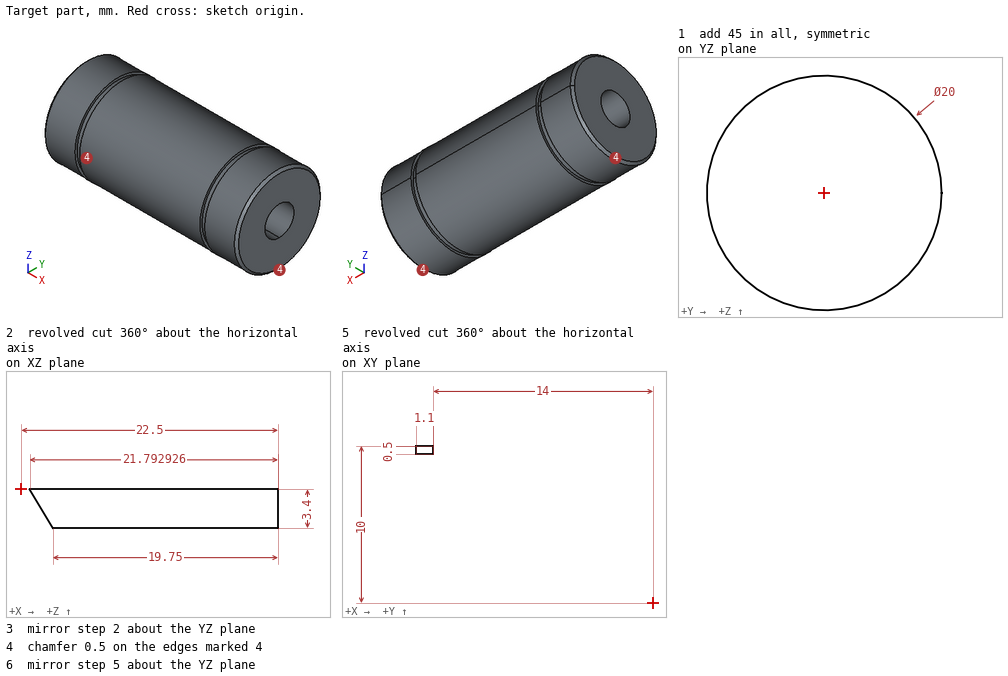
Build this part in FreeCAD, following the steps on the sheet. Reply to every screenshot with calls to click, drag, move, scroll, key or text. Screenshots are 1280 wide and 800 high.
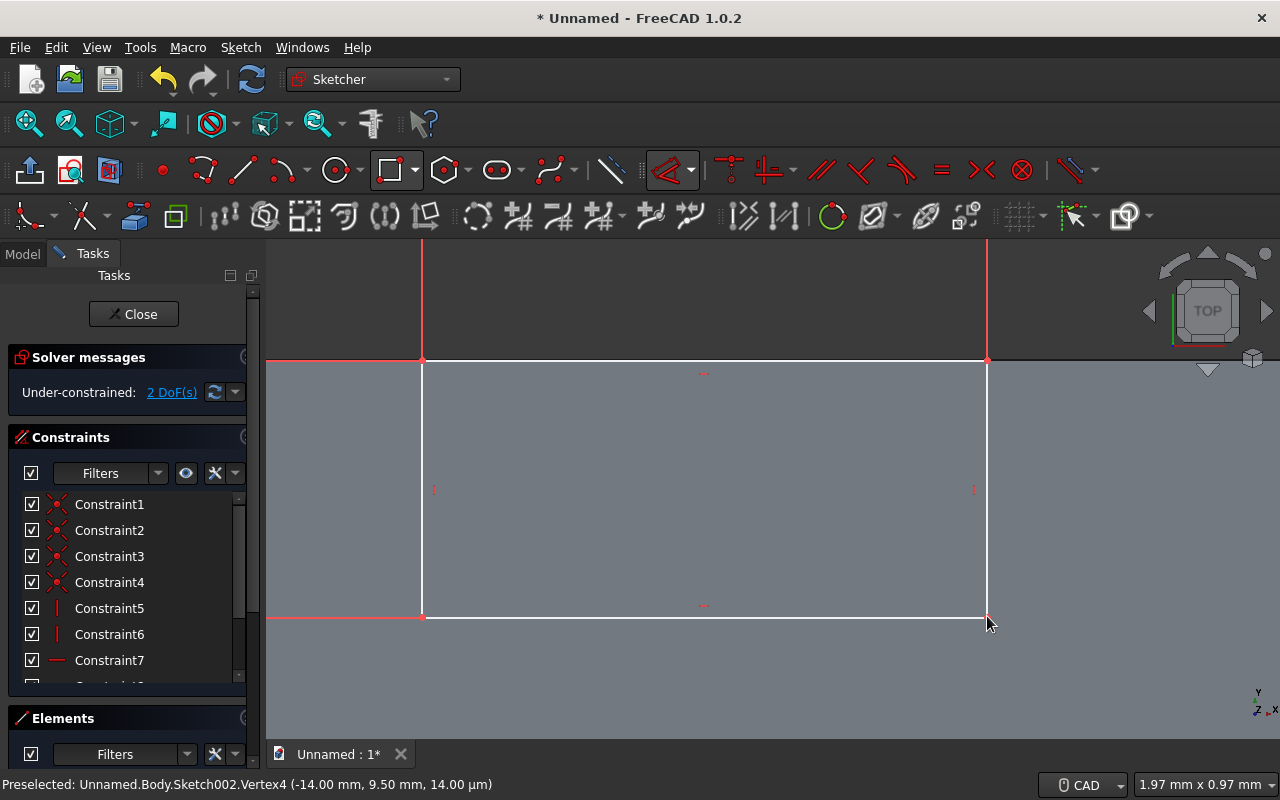
click(422, 361)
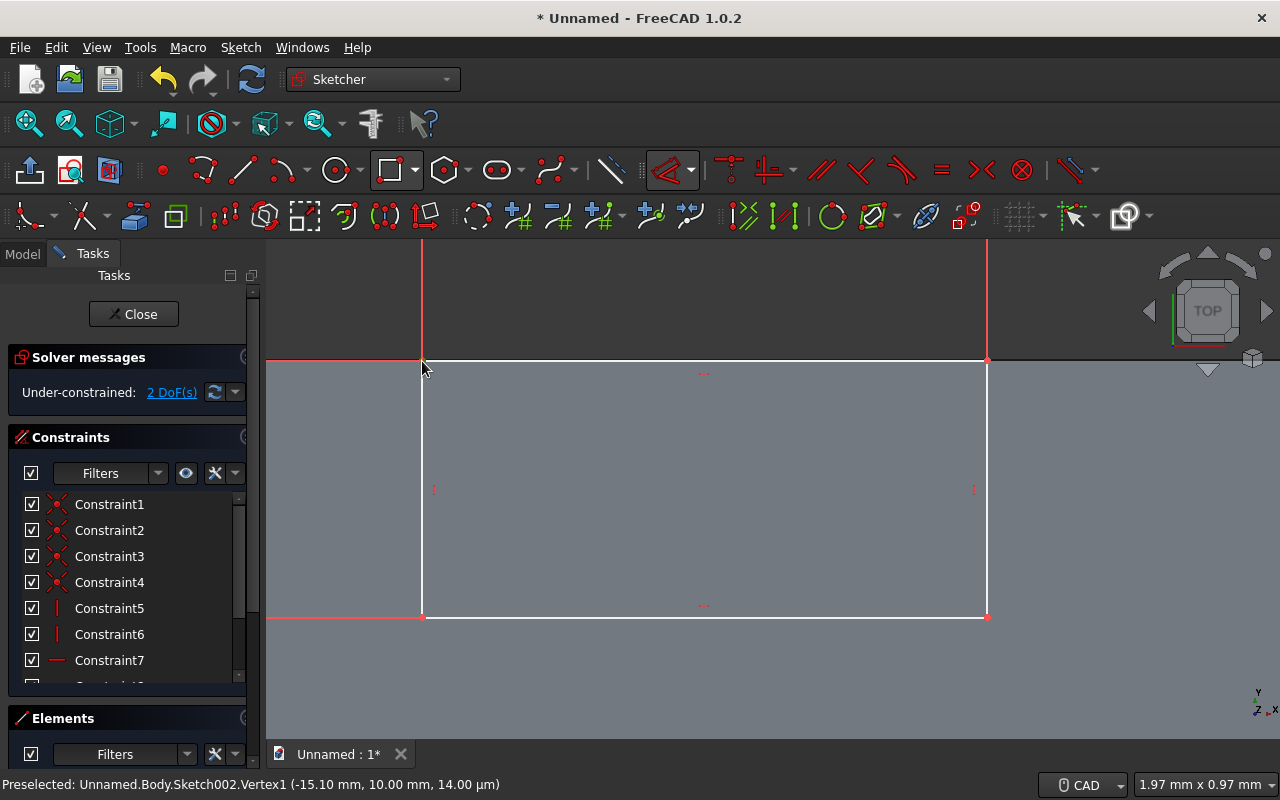
key(i)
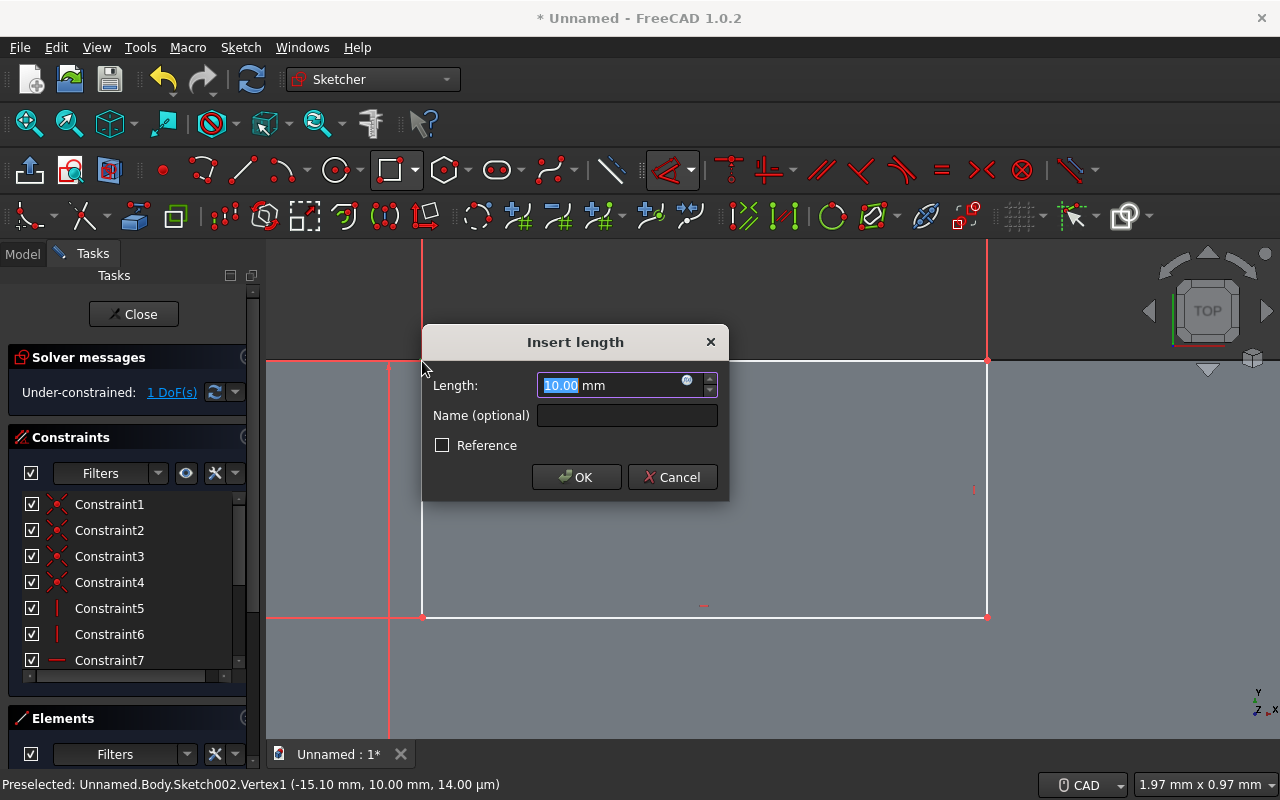
text(10)
key(Return)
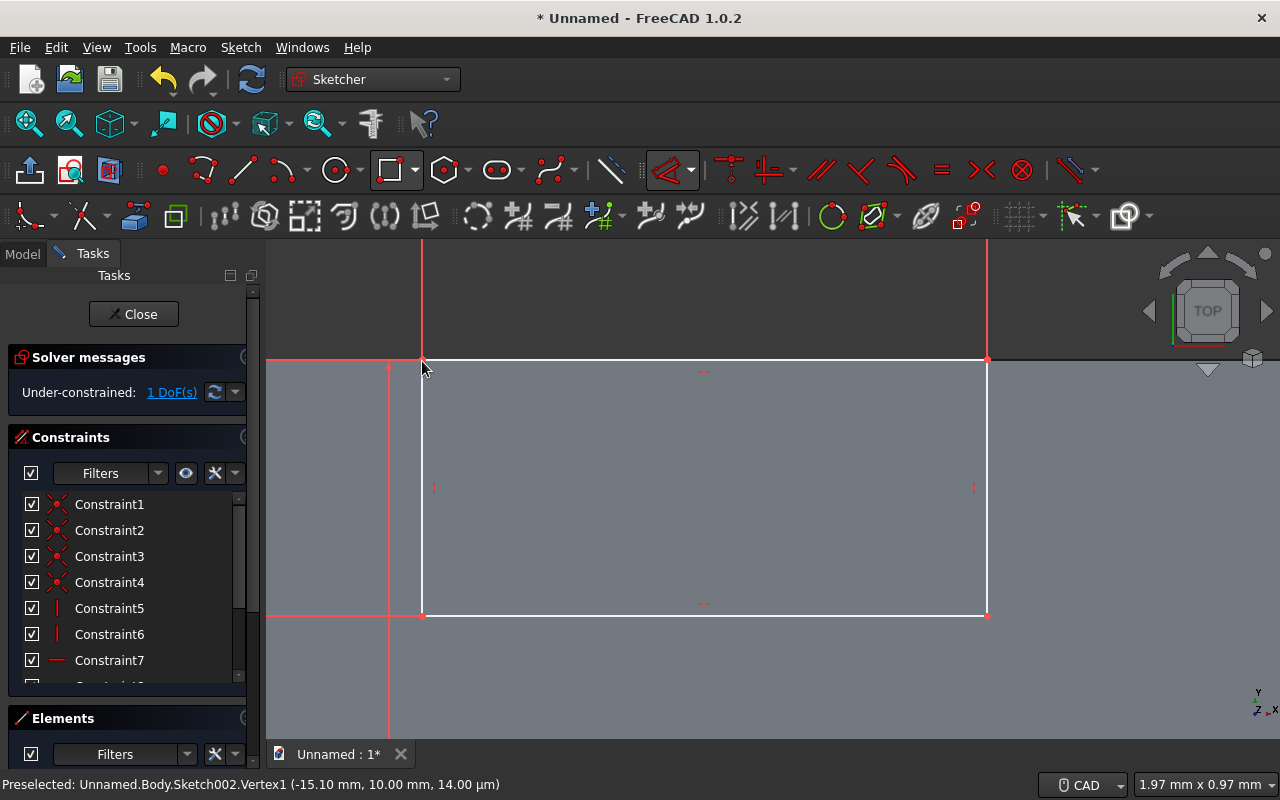
click(987, 616)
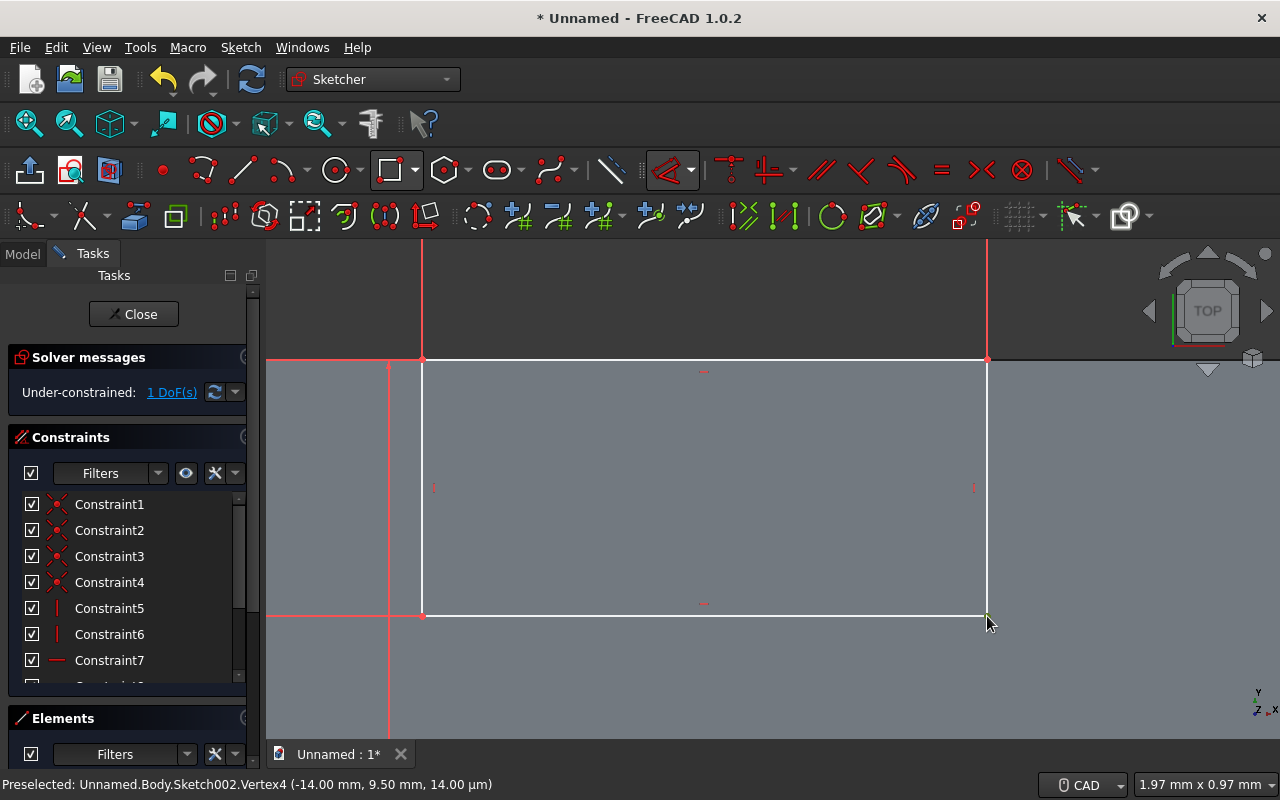
key(l)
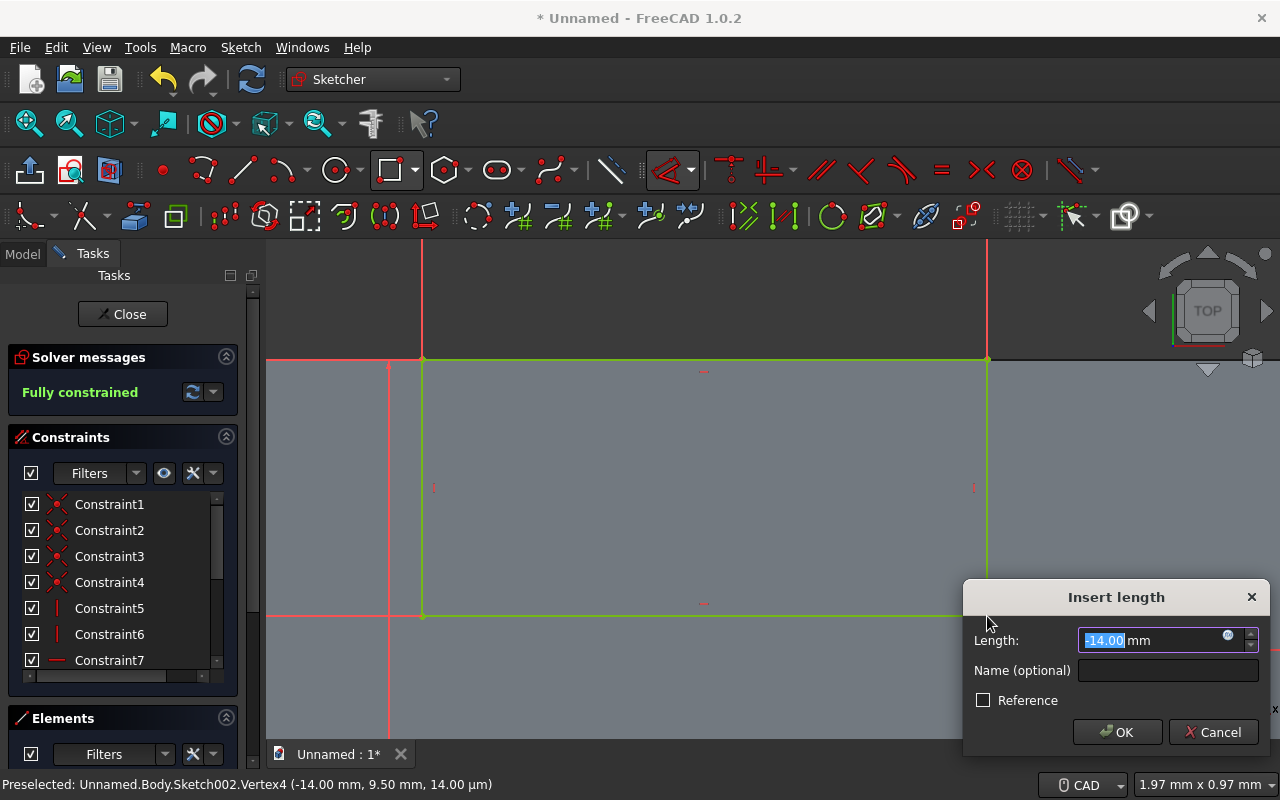
text(-14)
key(Return)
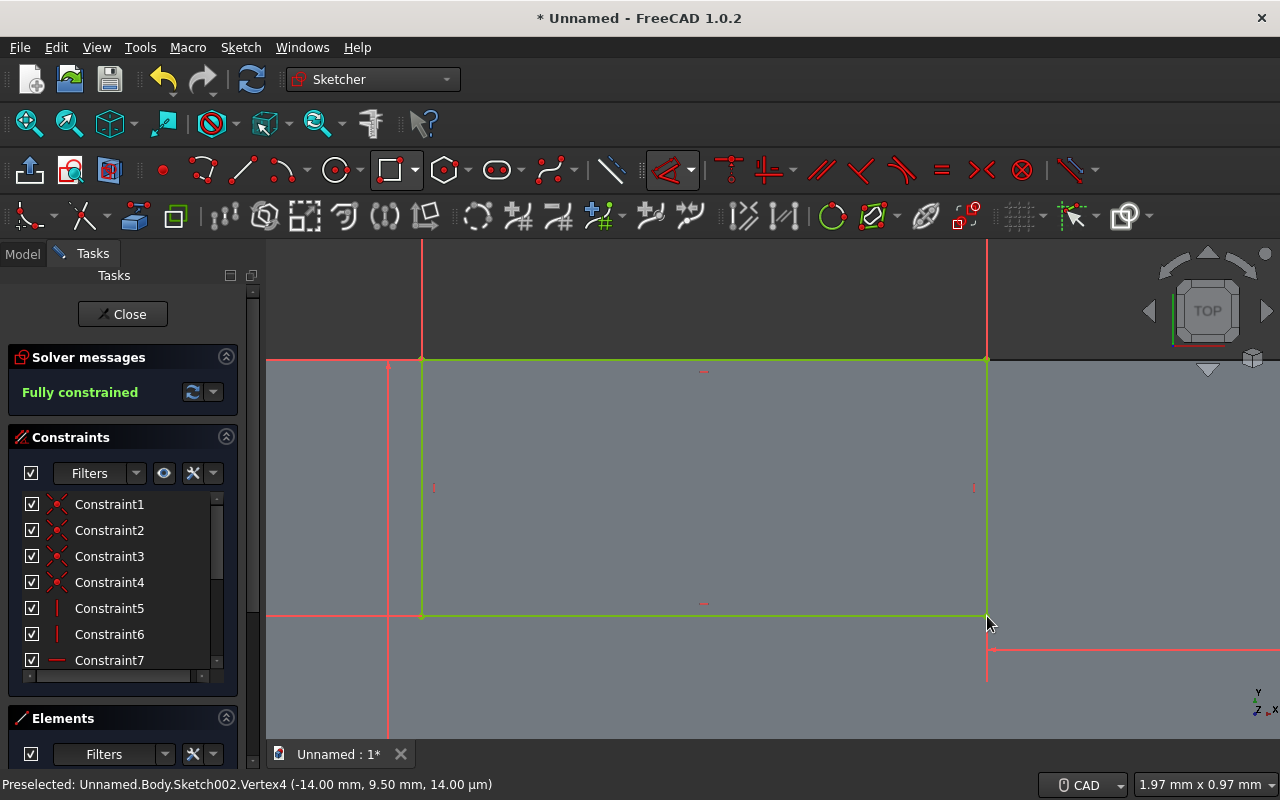
click(123, 314)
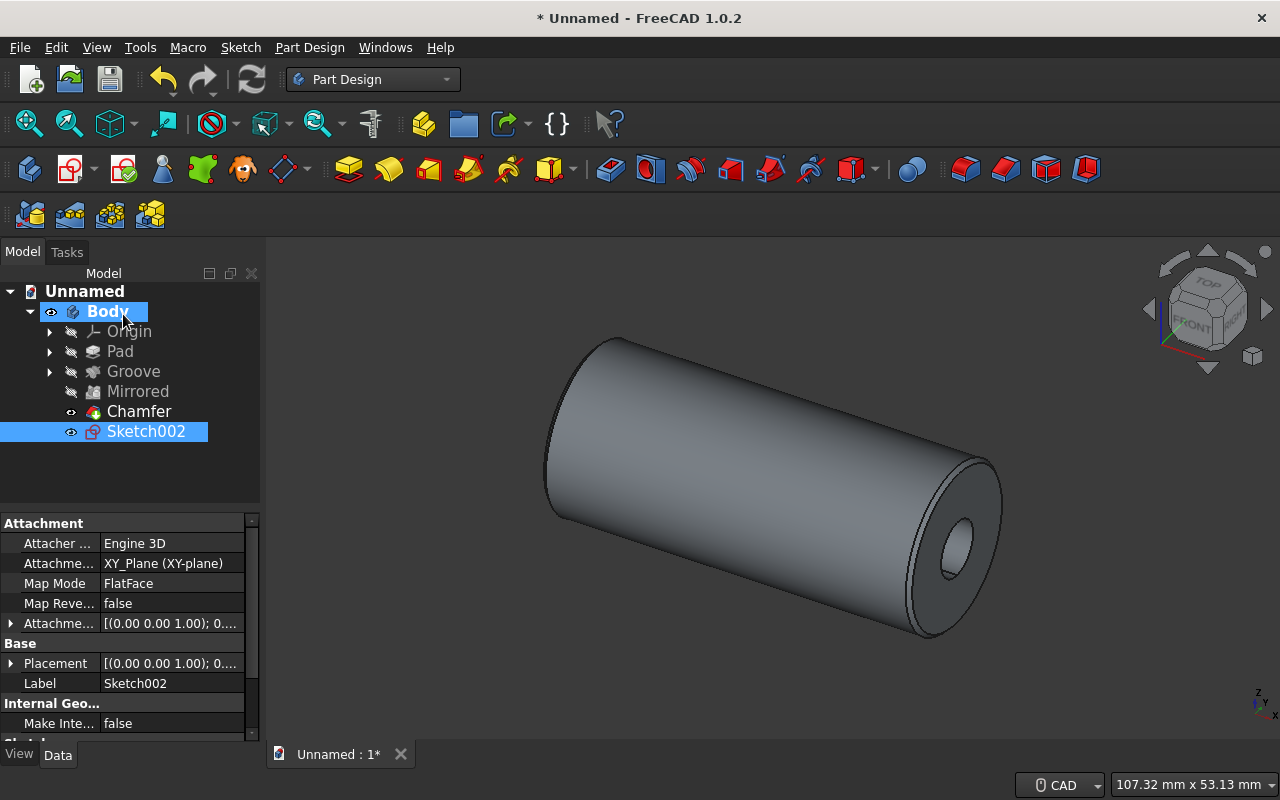
click(692, 170)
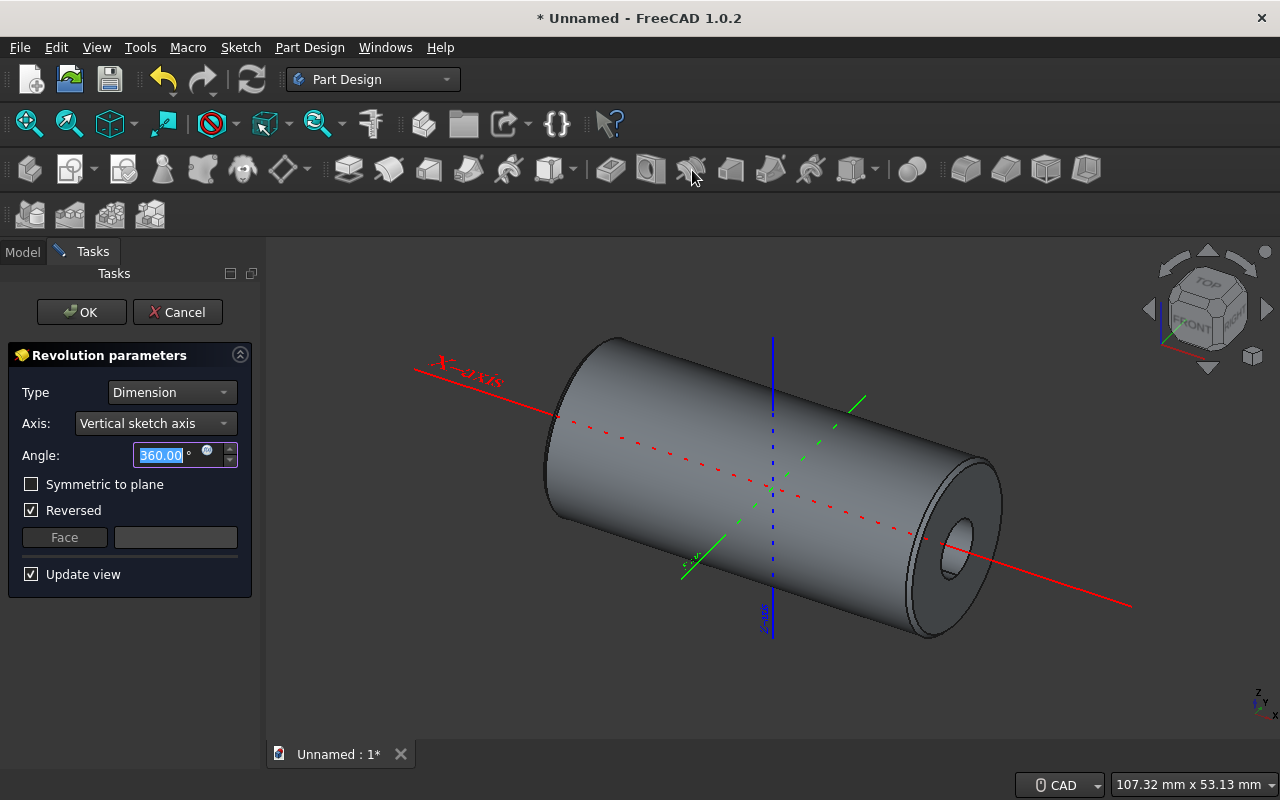
click(156, 424)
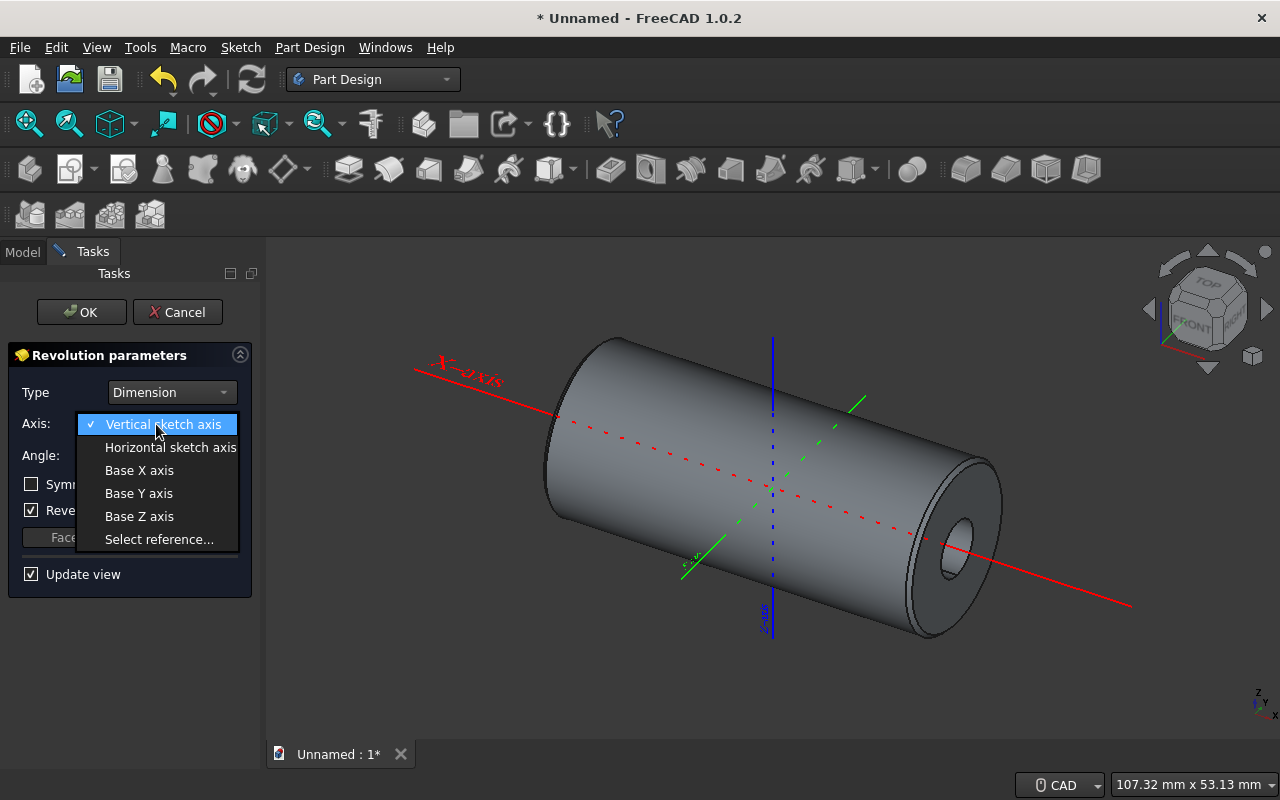
click(156, 448)